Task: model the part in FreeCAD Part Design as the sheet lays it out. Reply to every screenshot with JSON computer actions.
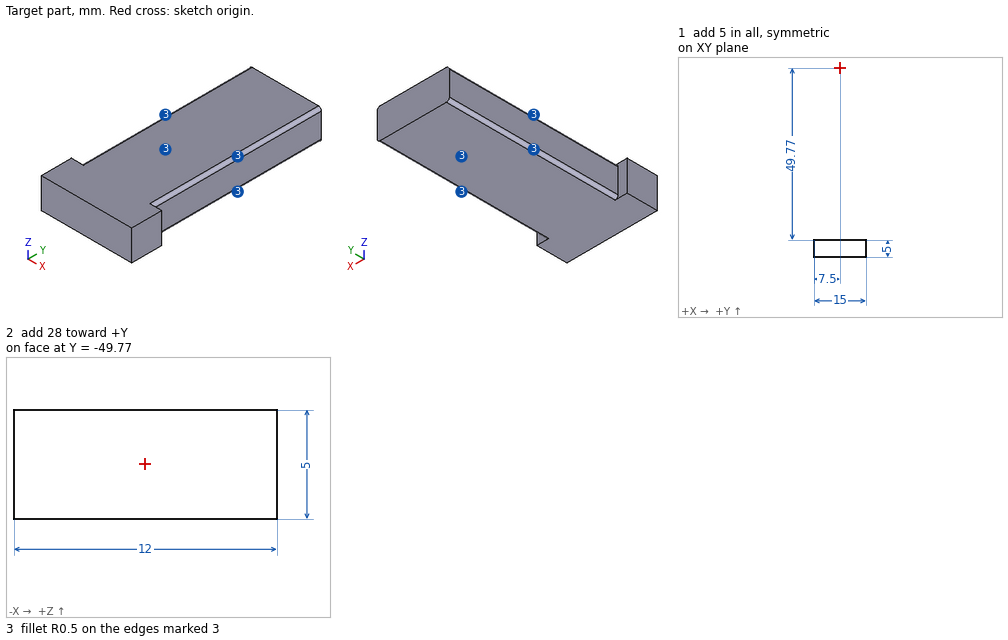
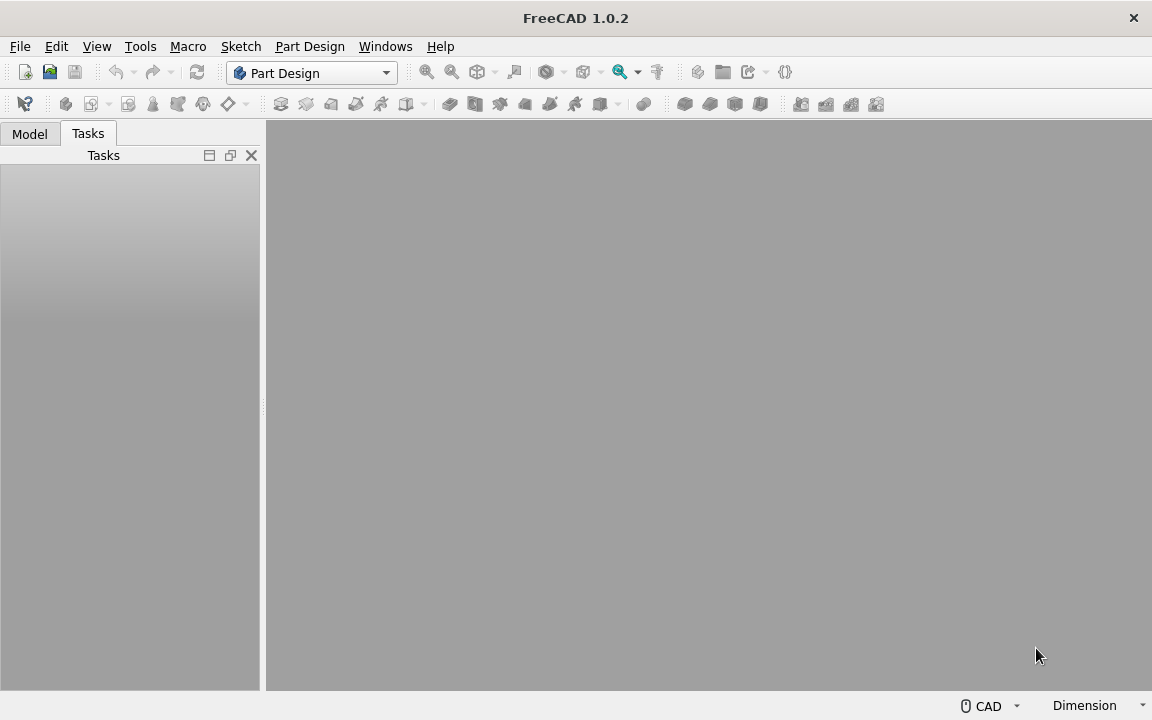
{"action": "left_click", "coordinate": [25, 72]}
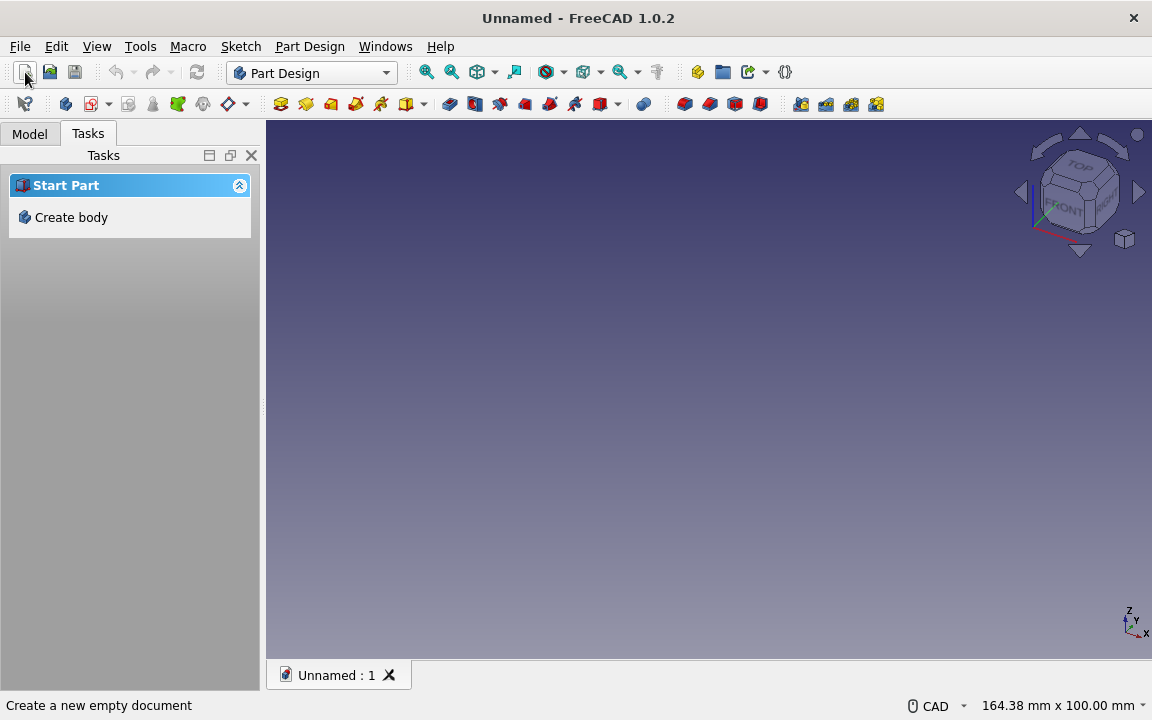
{"action": "left_click", "coordinate": [90, 104]}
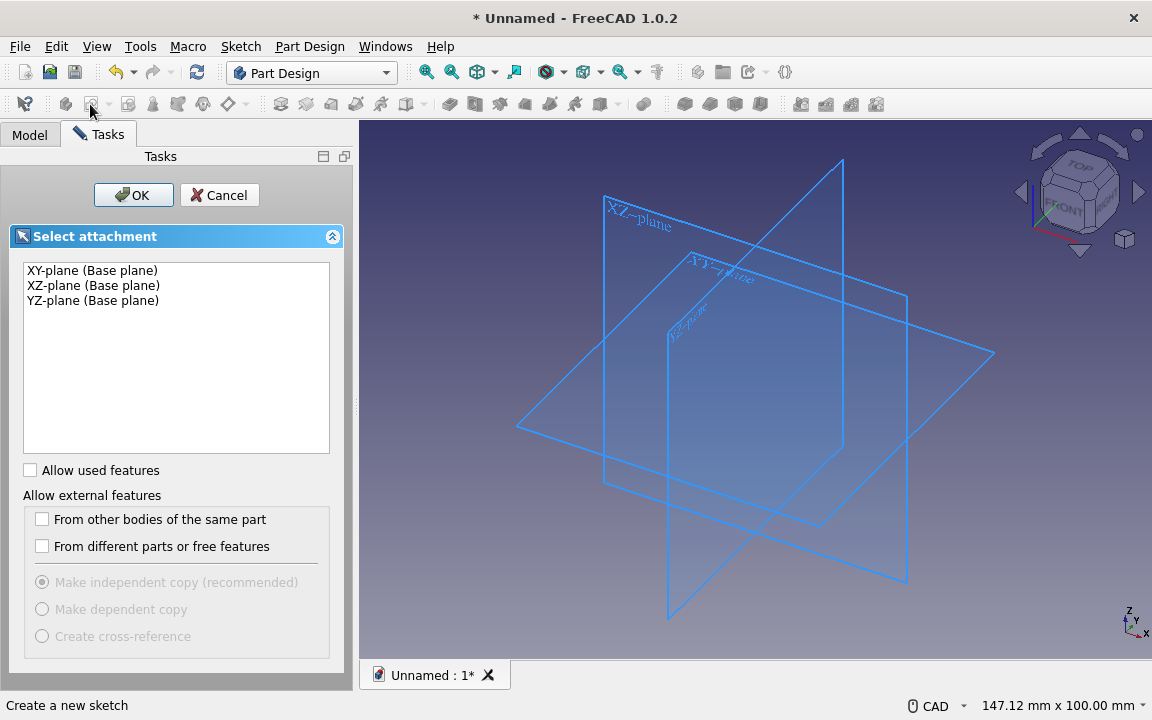
{"action": "left_click", "coordinate": [84, 270]}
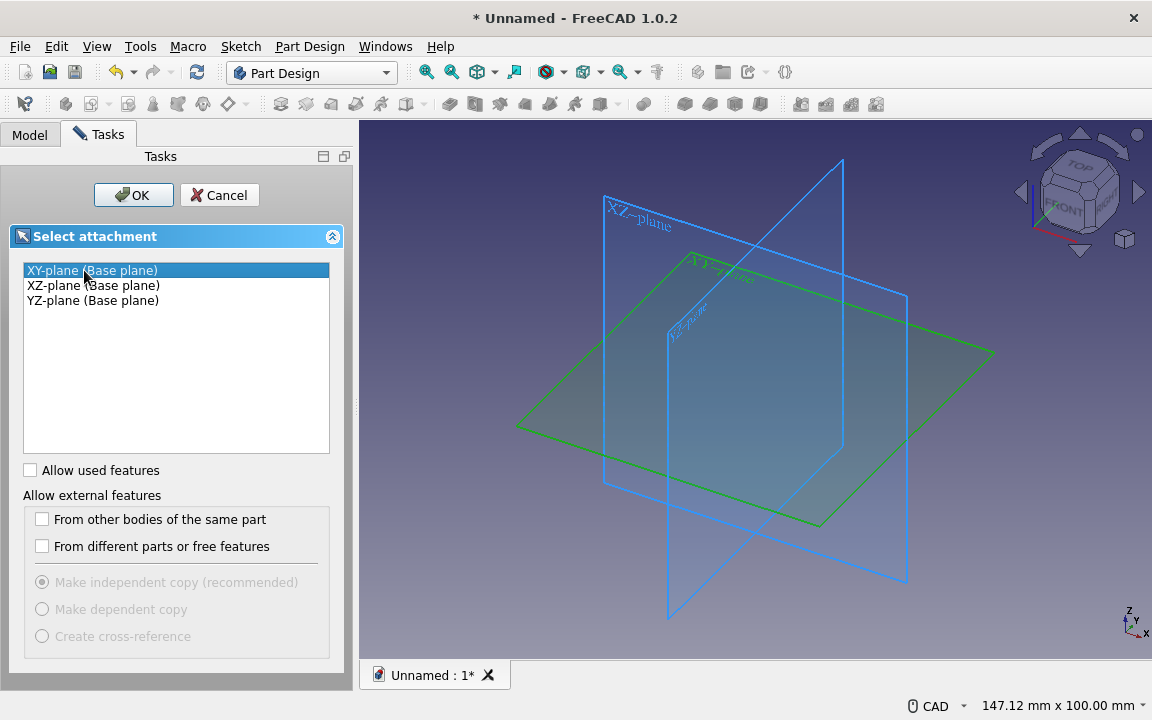
{"action": "left_click", "coordinate": [134, 195]}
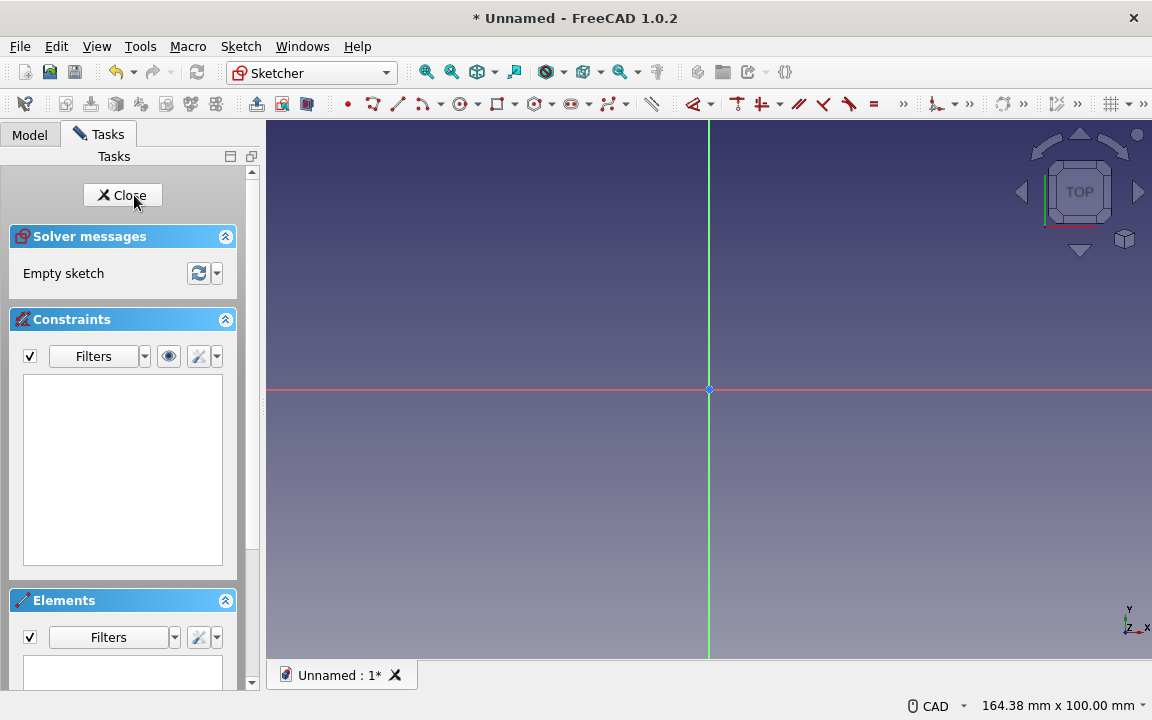
{"action": "scroll", "coordinate": [640, 390], "scroll_direction": "down", "scroll_amount": 5}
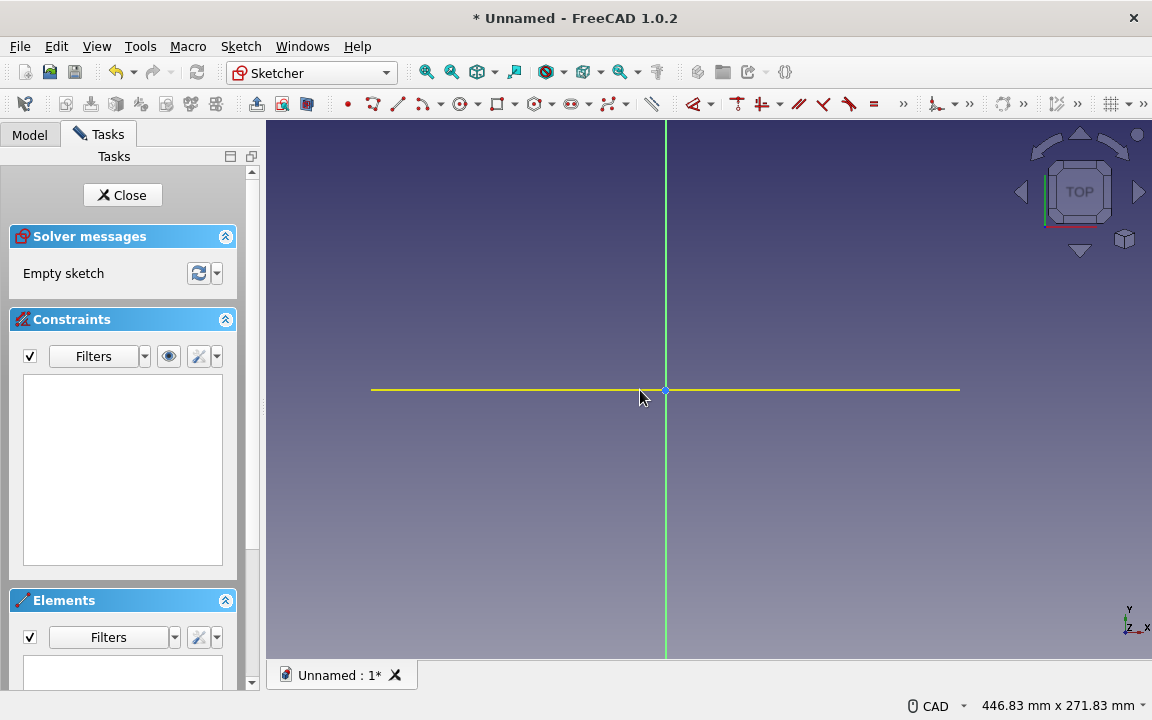
{"action": "scroll", "coordinate": [667, 501], "scroll_direction": "up", "scroll_amount": 14}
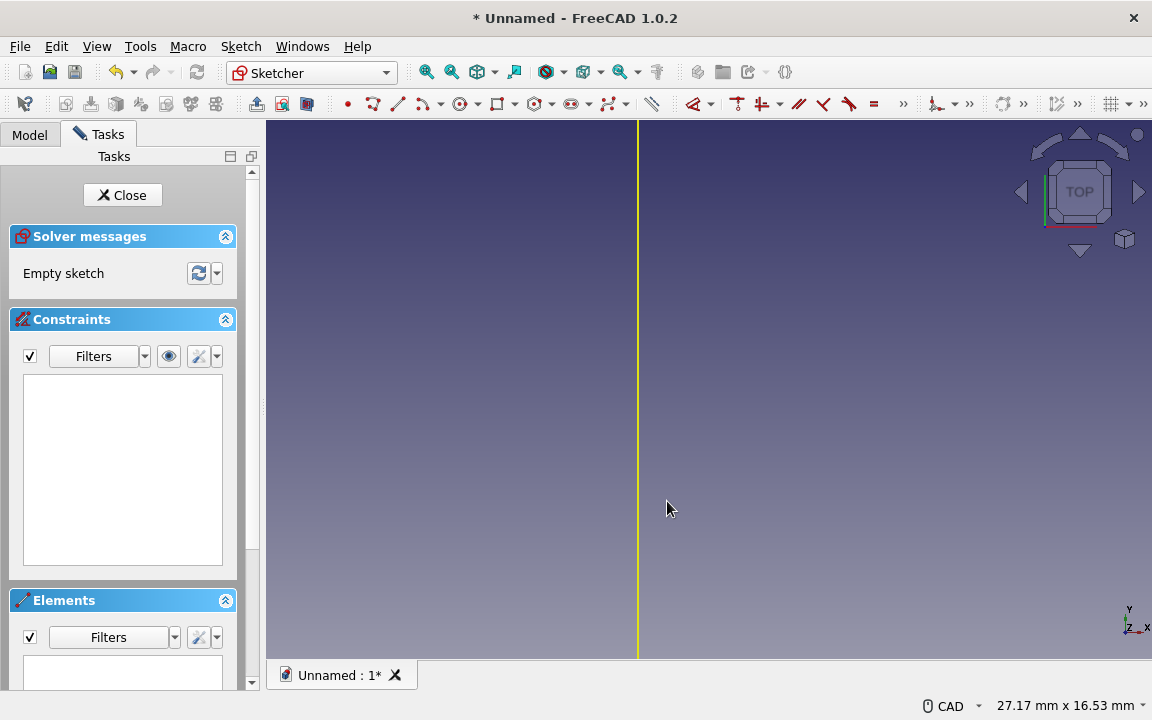
{"action": "left_click", "coordinate": [496, 104]}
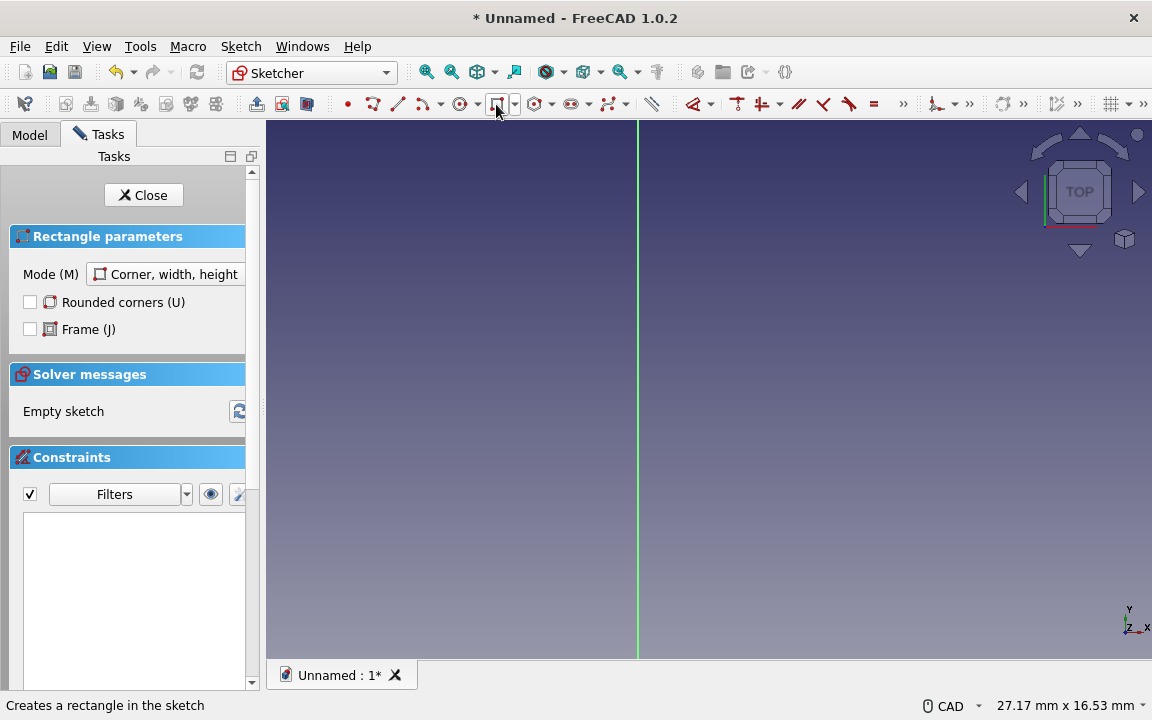
{"action": "left_click", "coordinate": [393, 290]}
{"action": "mouse_move", "coordinate": [882, 453]}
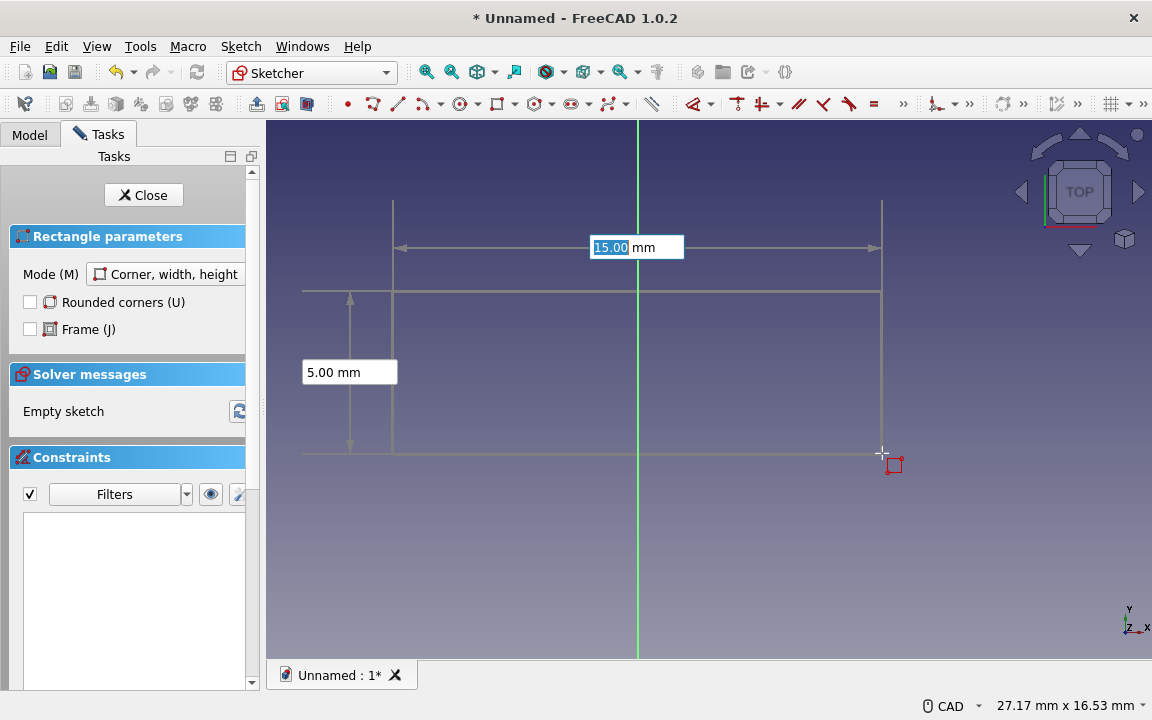
{"action": "type", "text": "15"}
{"action": "key", "text": "Tab"}
{"action": "type", "text": "5"}
{"action": "key", "text": "Return"}
{"action": "key", "text": "Escape"}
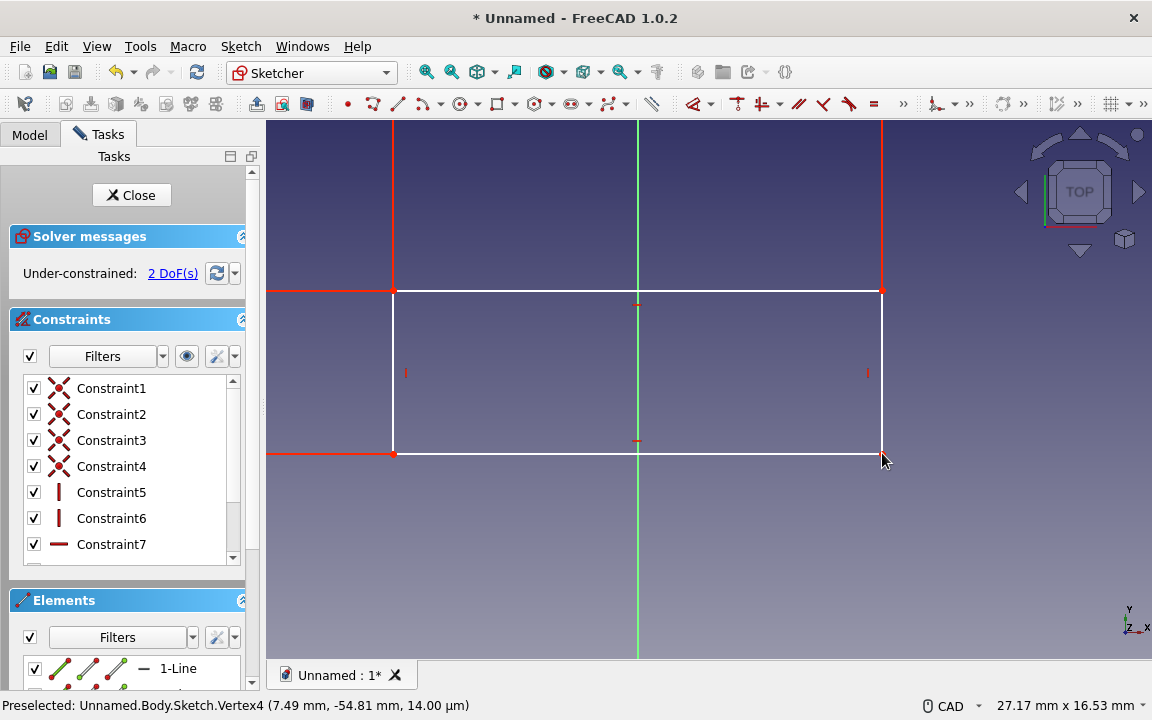
{"action": "left_click", "coordinate": [692, 104]}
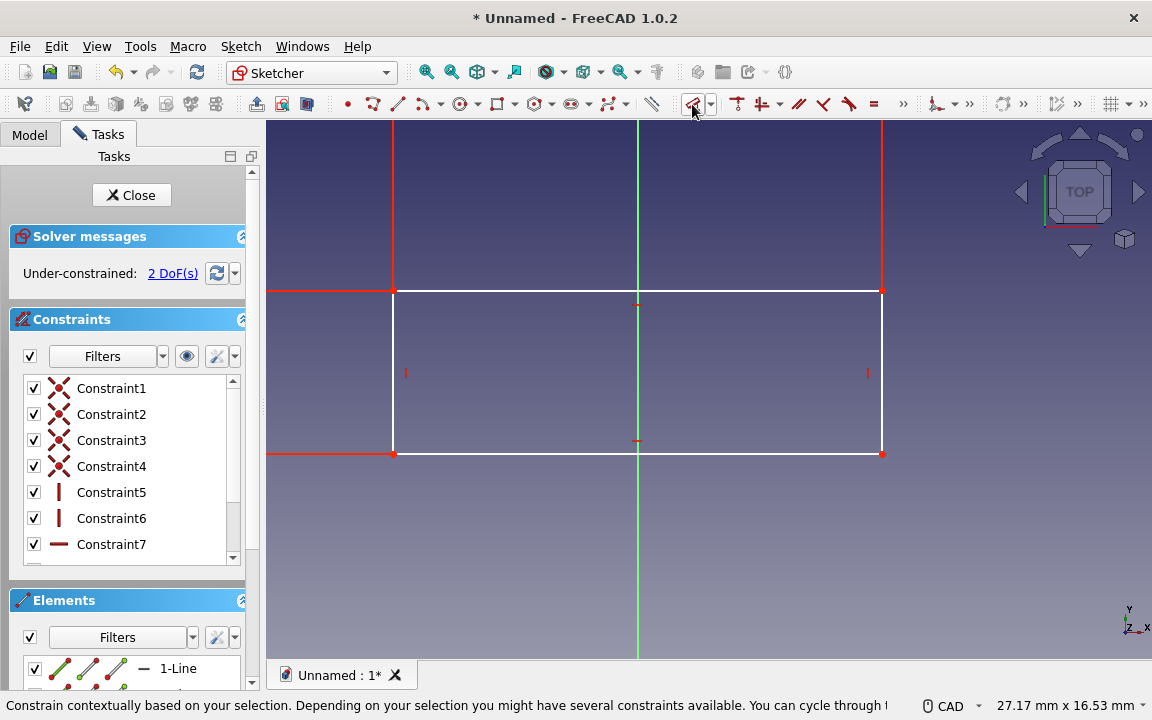
{"action": "left_click", "coordinate": [393, 291]}
{"action": "left_click", "coordinate": [515, 325]}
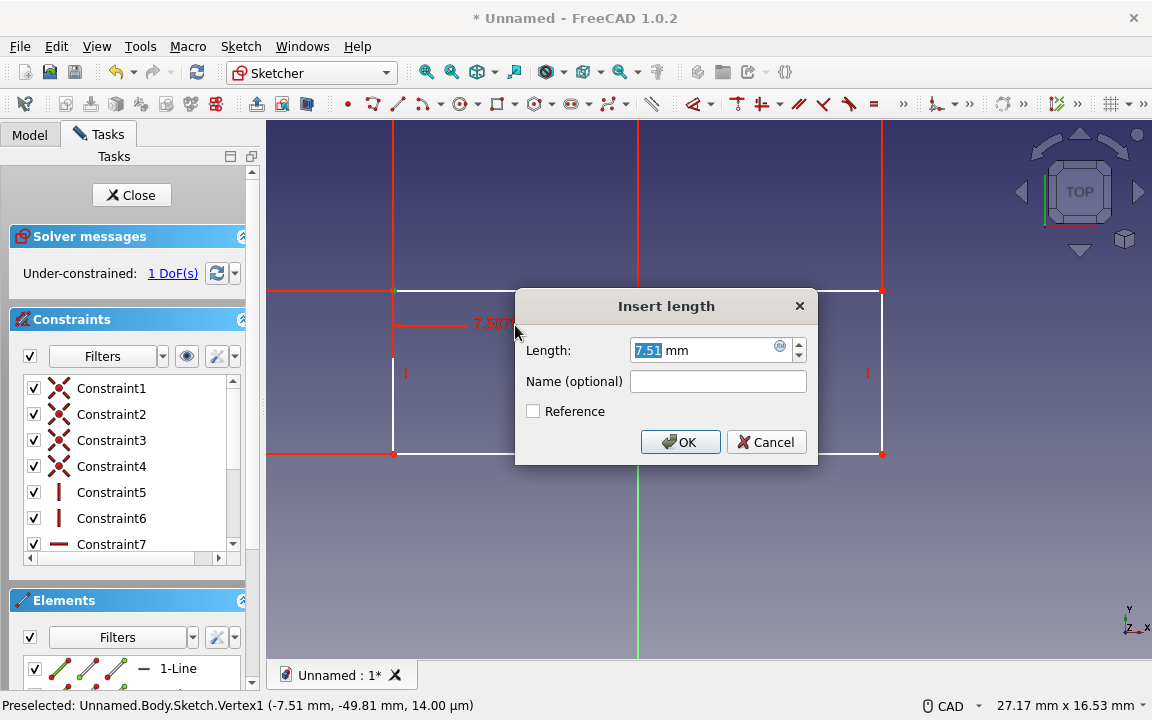
{"action": "type", "text": "7.5"}
{"action": "key", "text": "Return"}